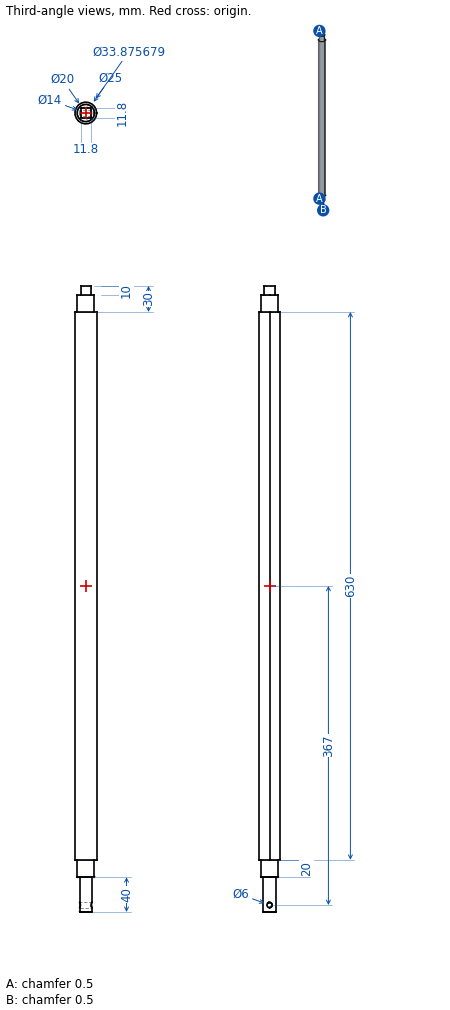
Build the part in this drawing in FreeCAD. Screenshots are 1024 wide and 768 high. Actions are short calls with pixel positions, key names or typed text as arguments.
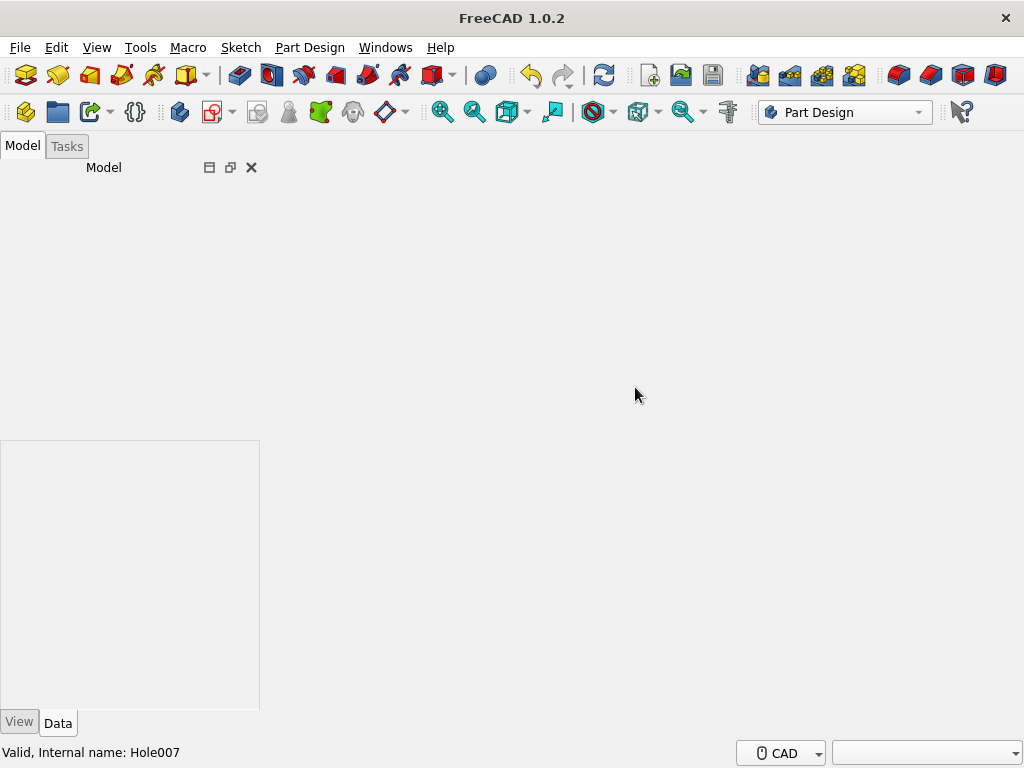
click(650, 76)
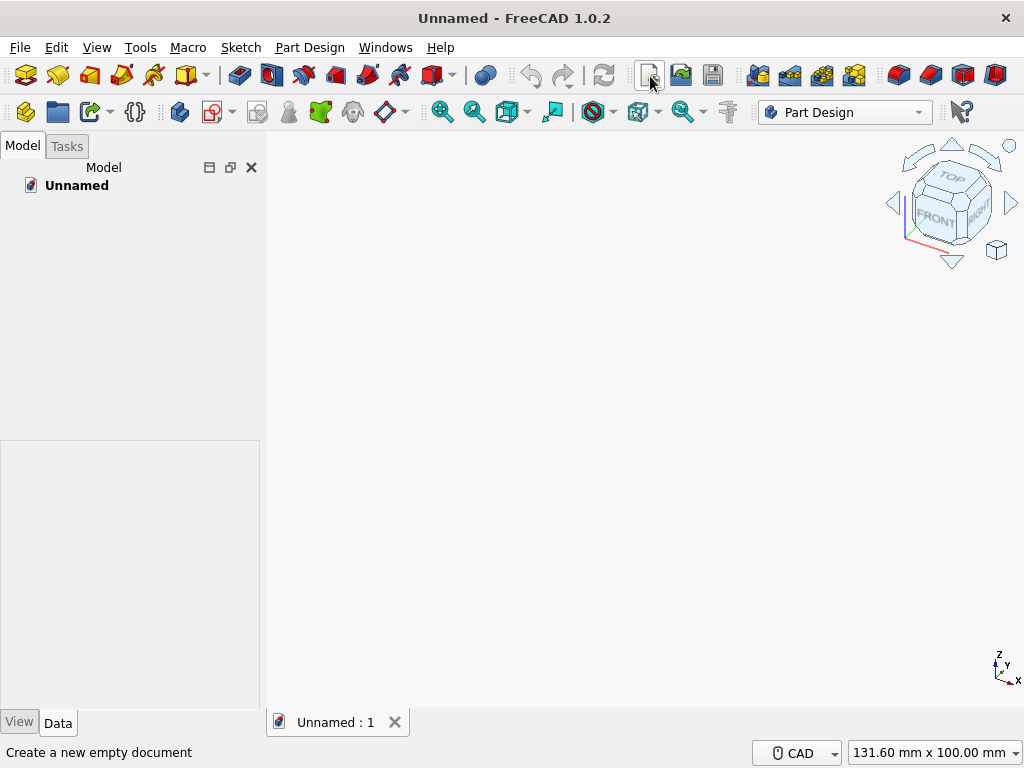
click(212, 112)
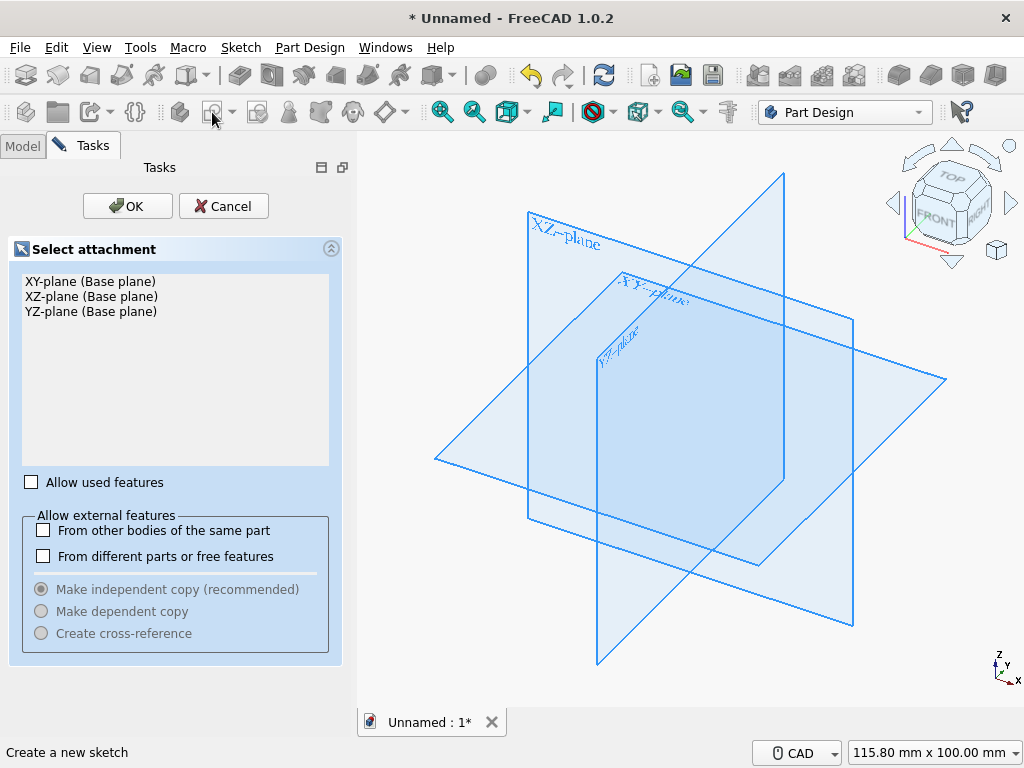
click(82, 282)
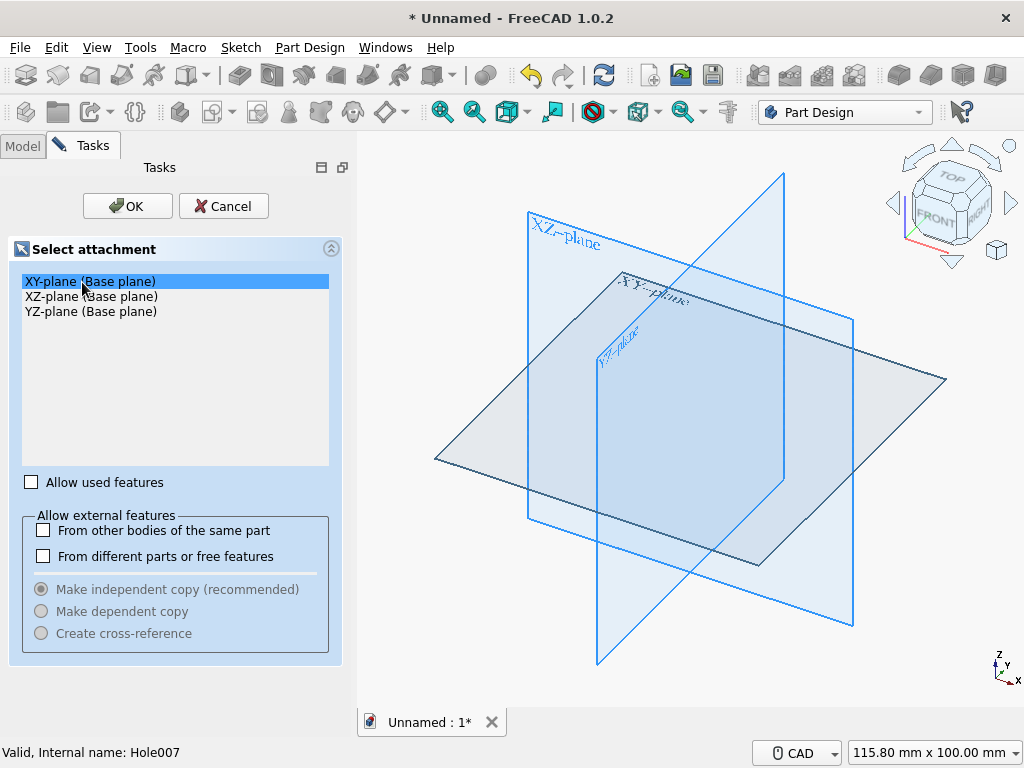
click(128, 206)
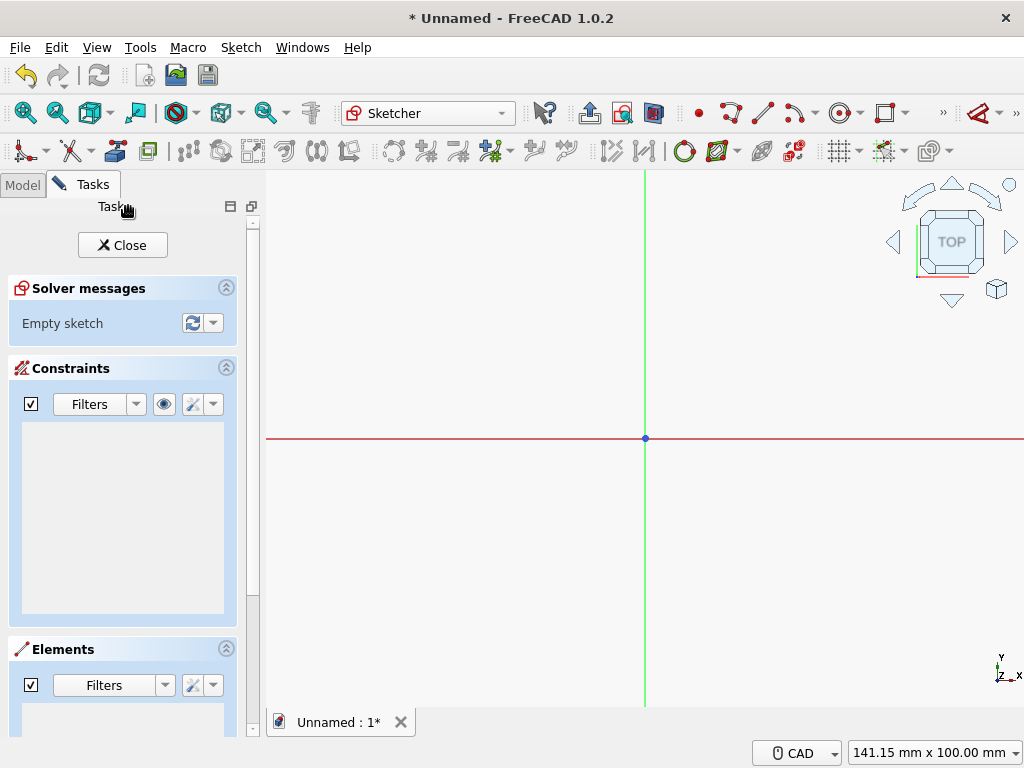
scroll(685, 439, up, 5)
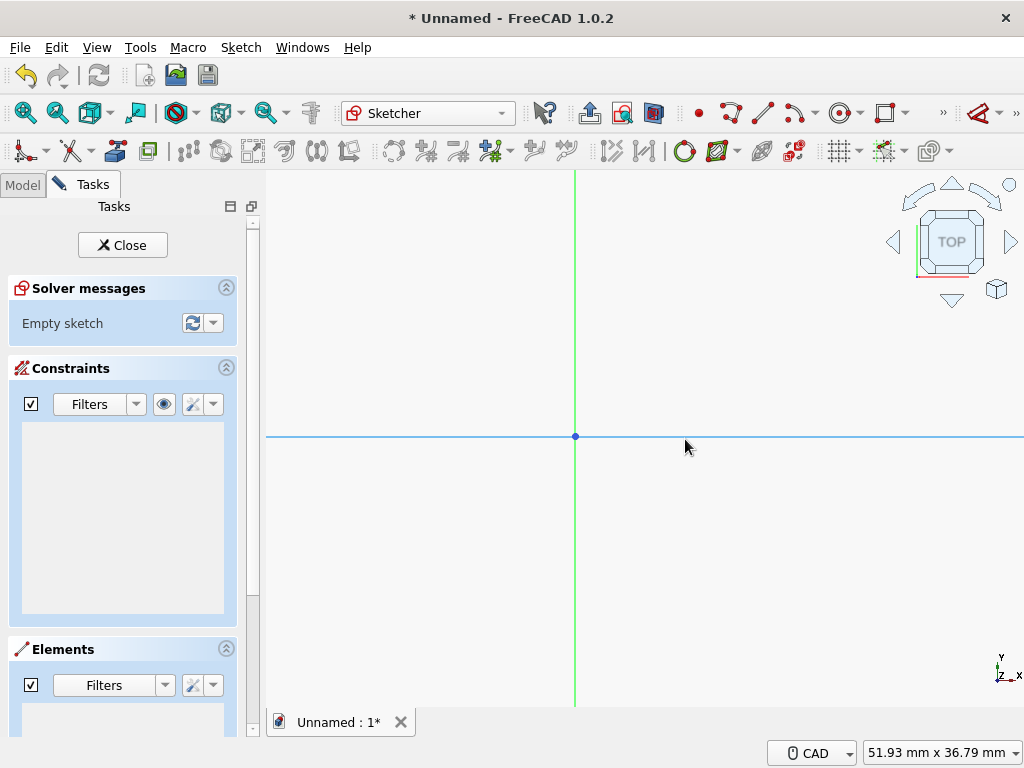
click(840, 114)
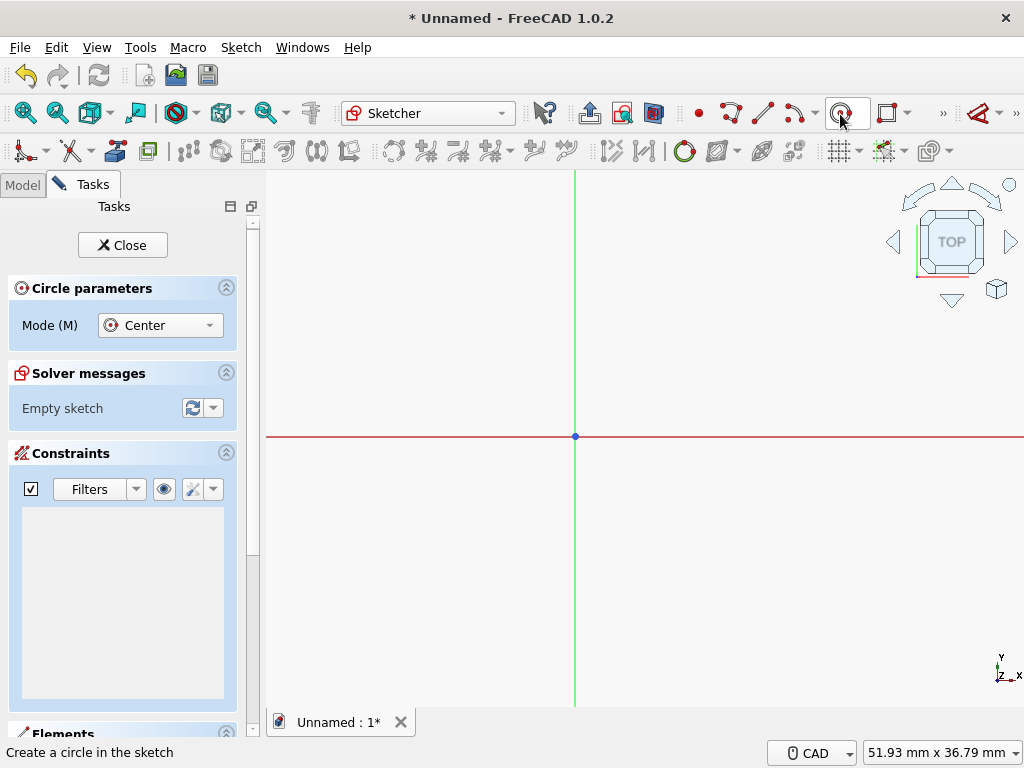
click(575, 437)
move(704, 308)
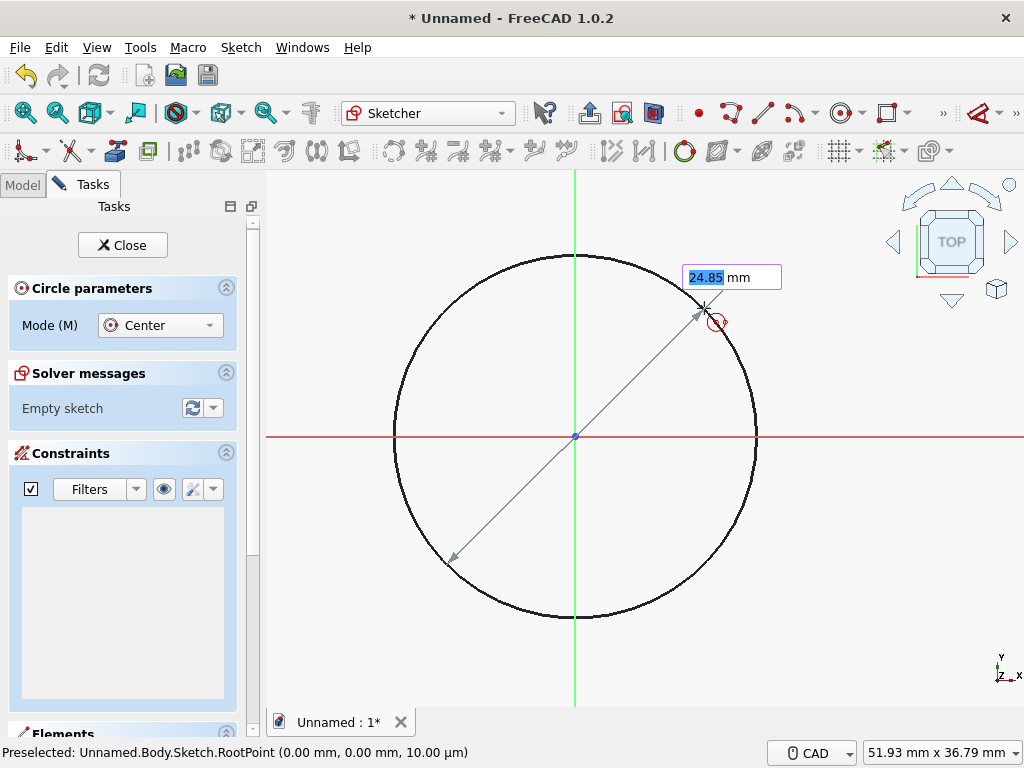
text(25)
key(Return)
key(Escape)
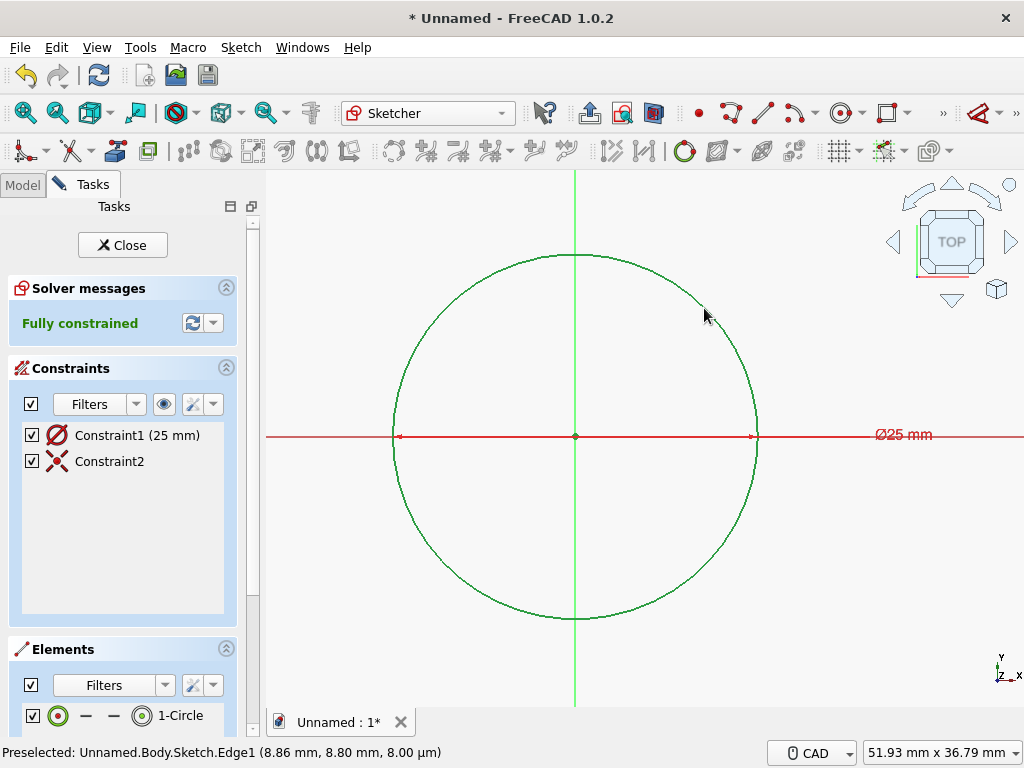
click(123, 245)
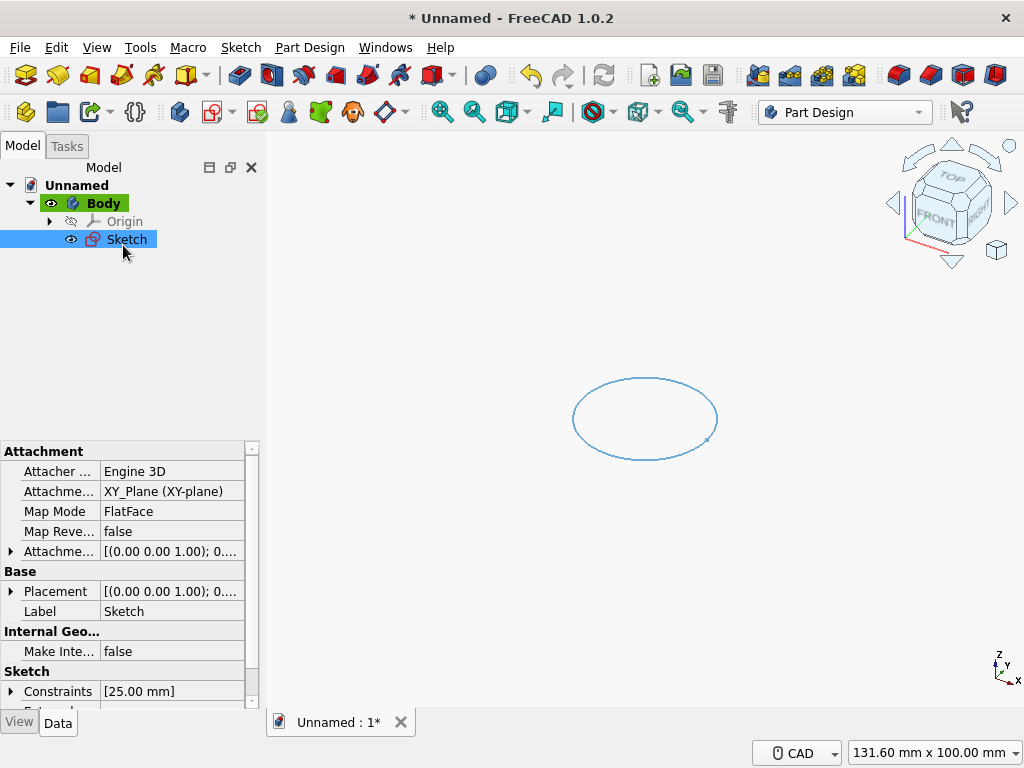
click(26, 76)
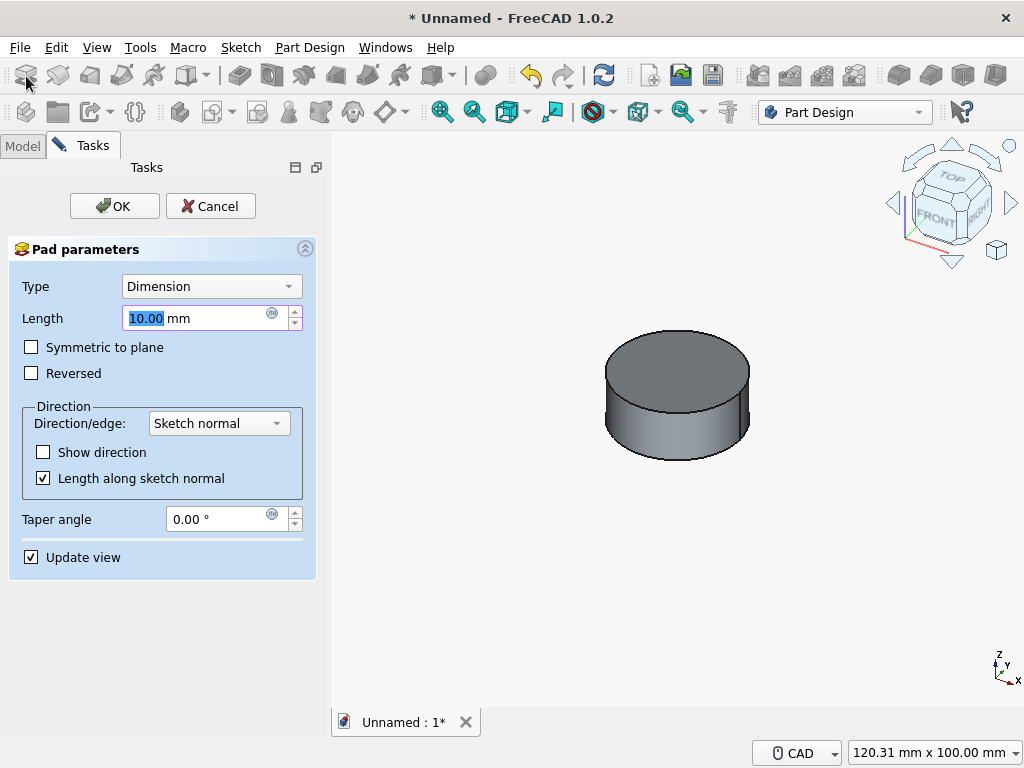
text(630)
key(Tab)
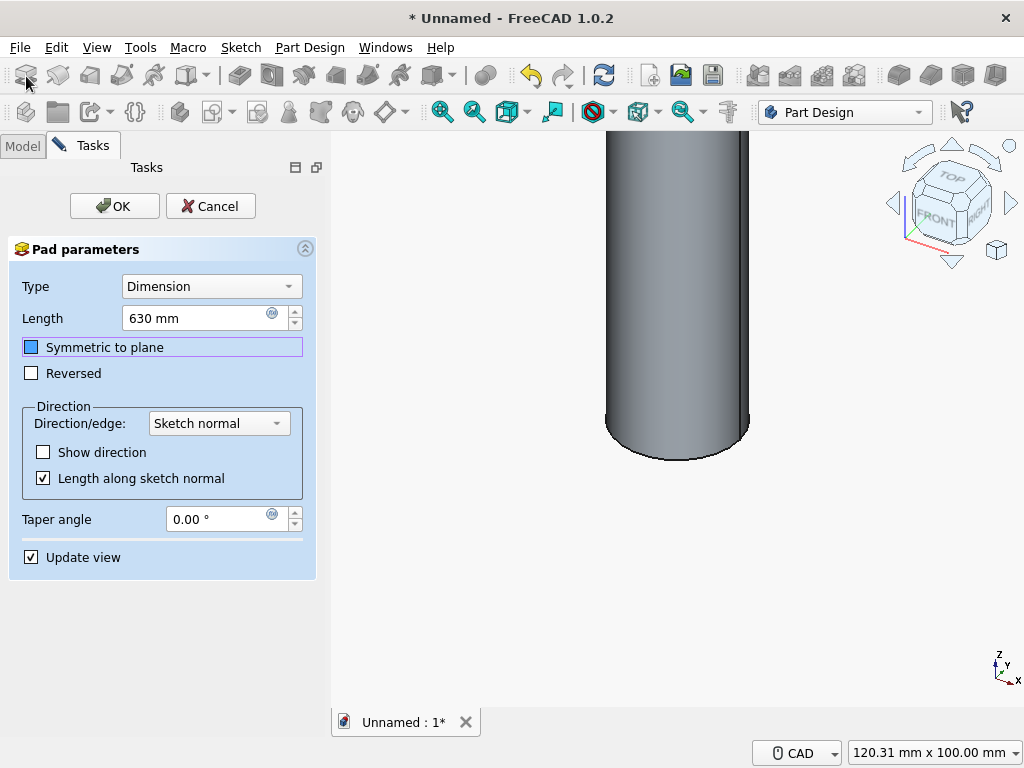
click(30, 347)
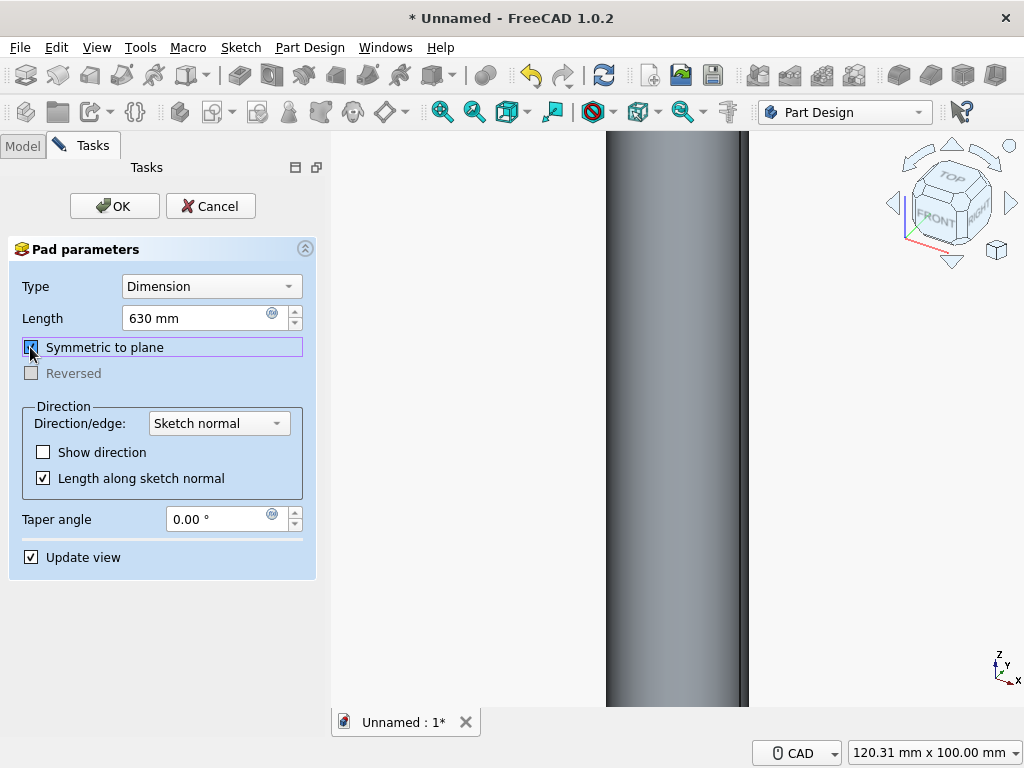
click(115, 206)